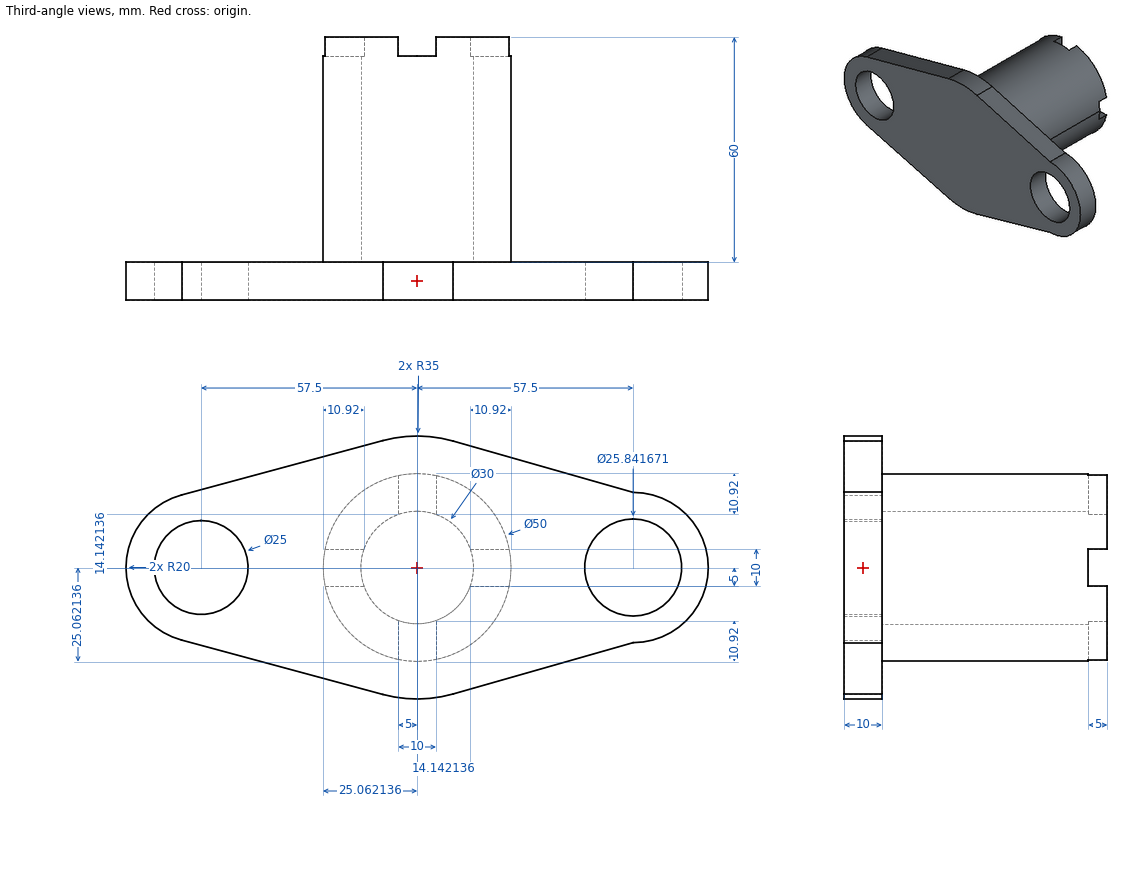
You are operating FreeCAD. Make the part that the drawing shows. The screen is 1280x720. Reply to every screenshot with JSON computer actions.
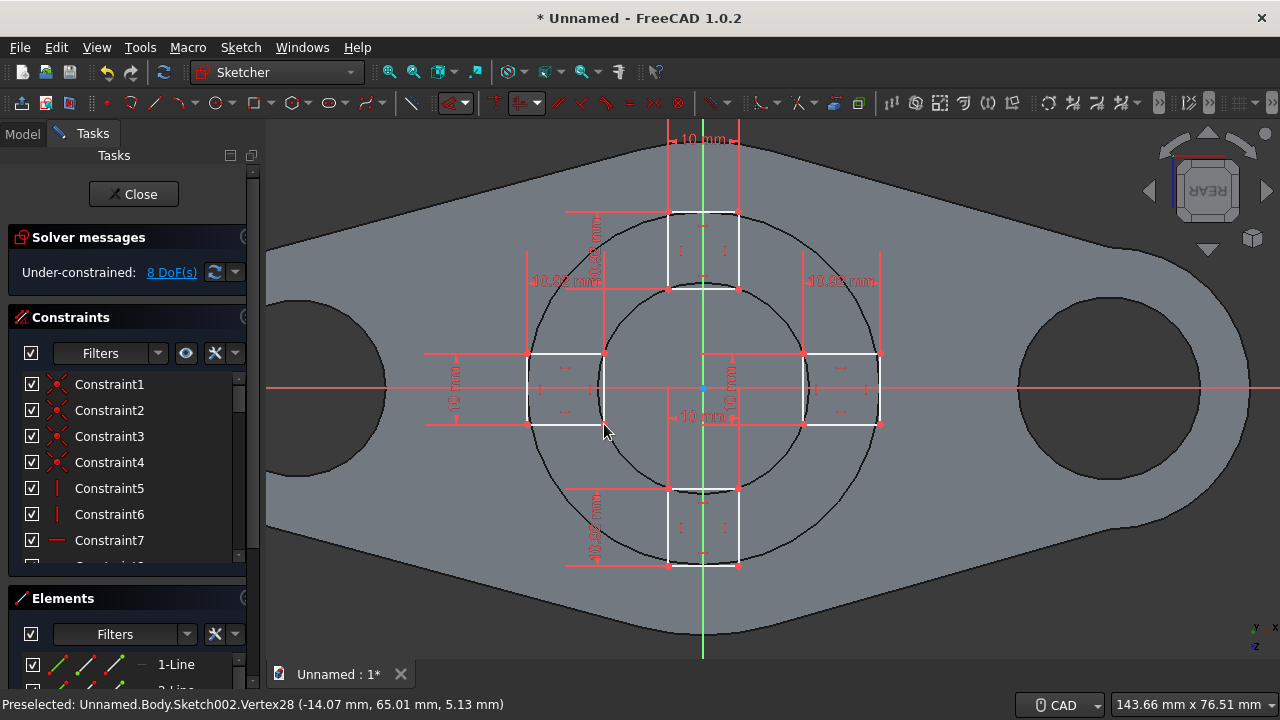
{"action": "left_click", "coordinate": [668, 212]}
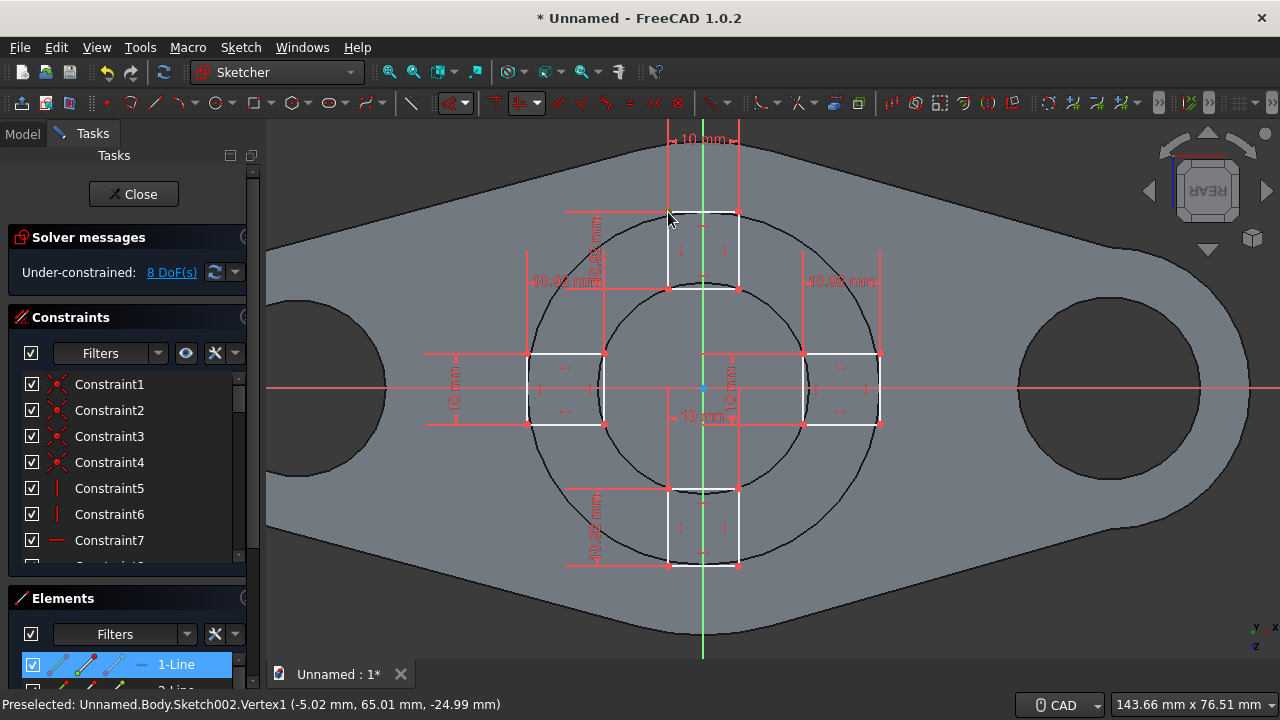
{"action": "left_click", "coordinate": [468, 104]}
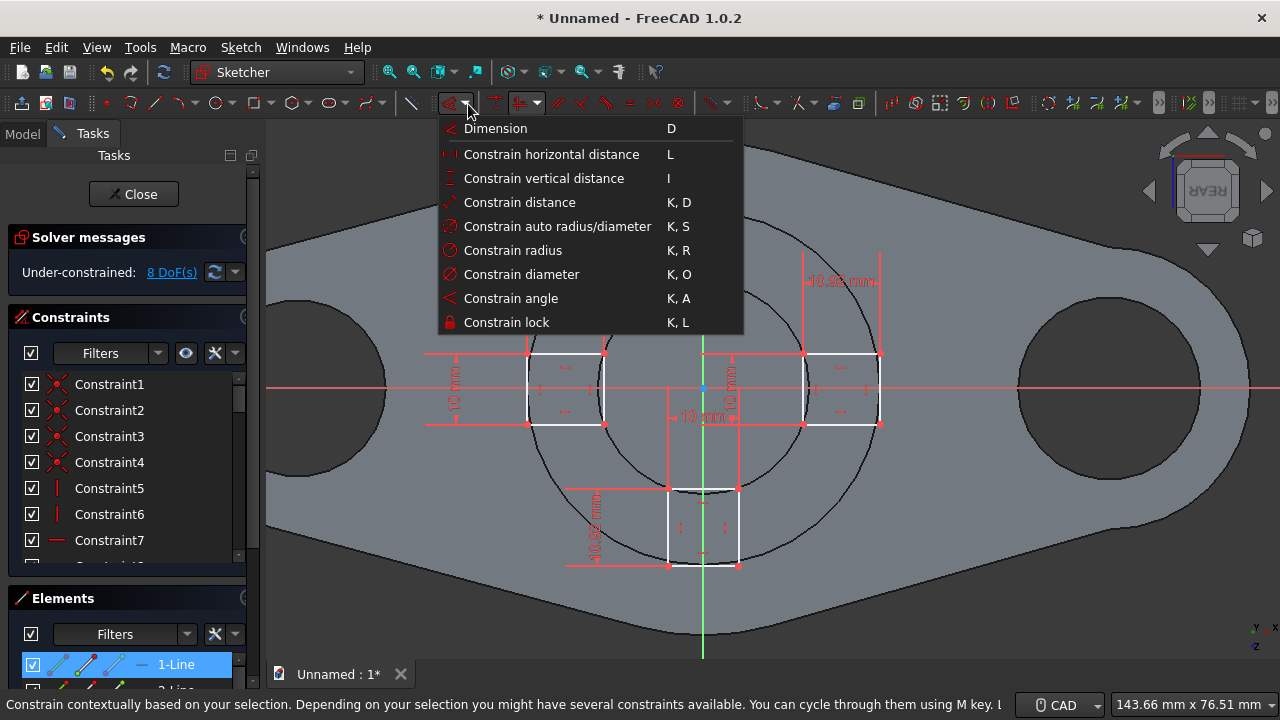
{"action": "left_click", "coordinate": [591, 154]}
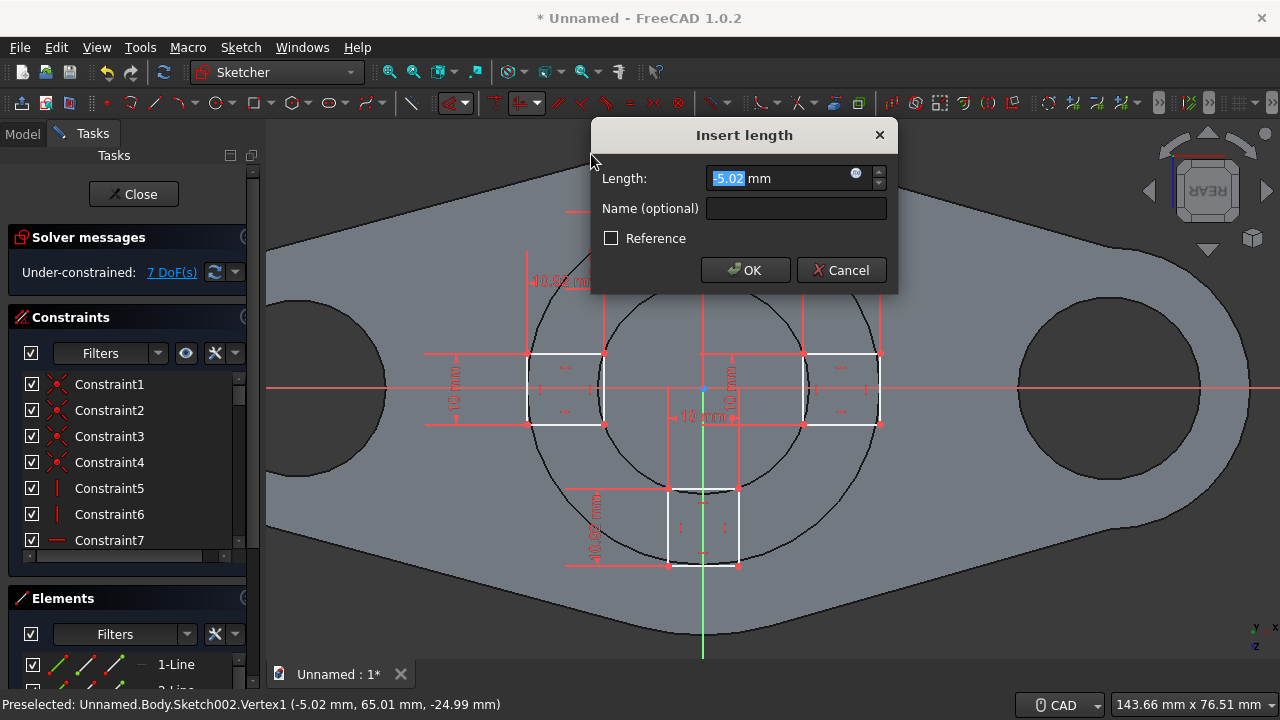
{"action": "type", "text": "-5"}
{"action": "key", "text": "Return"}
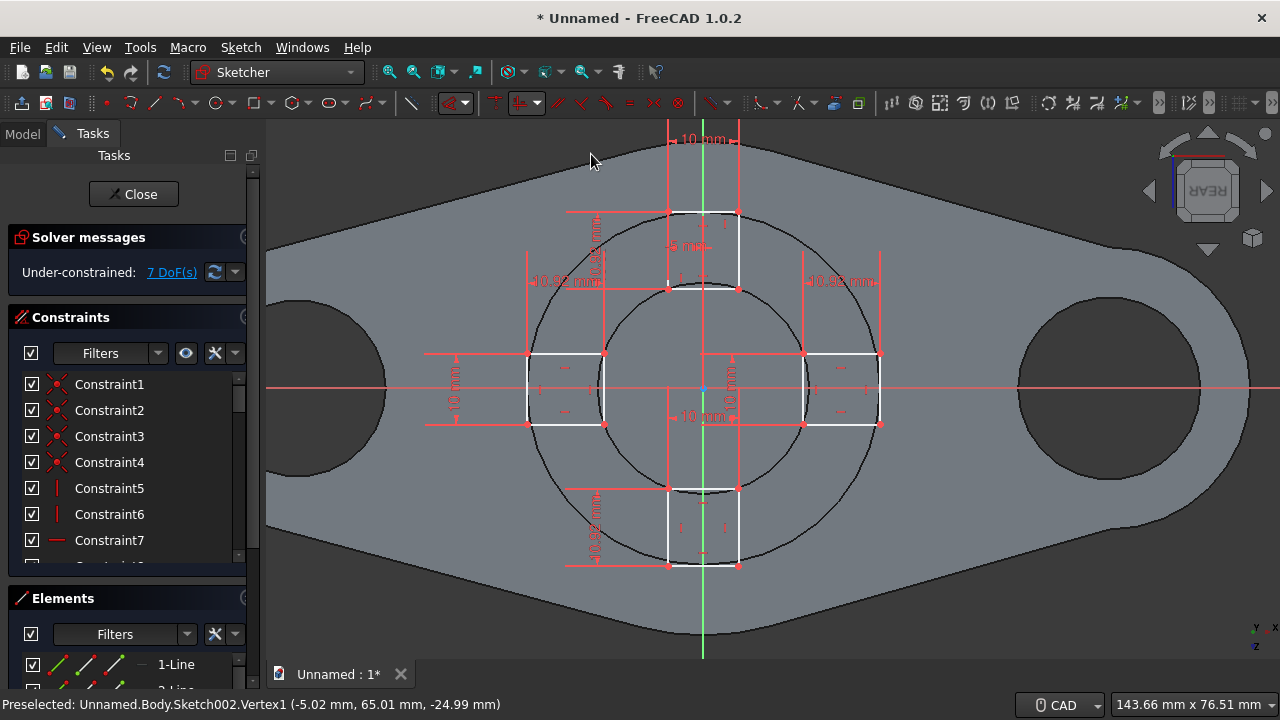
{"action": "left_click", "coordinate": [803, 354]}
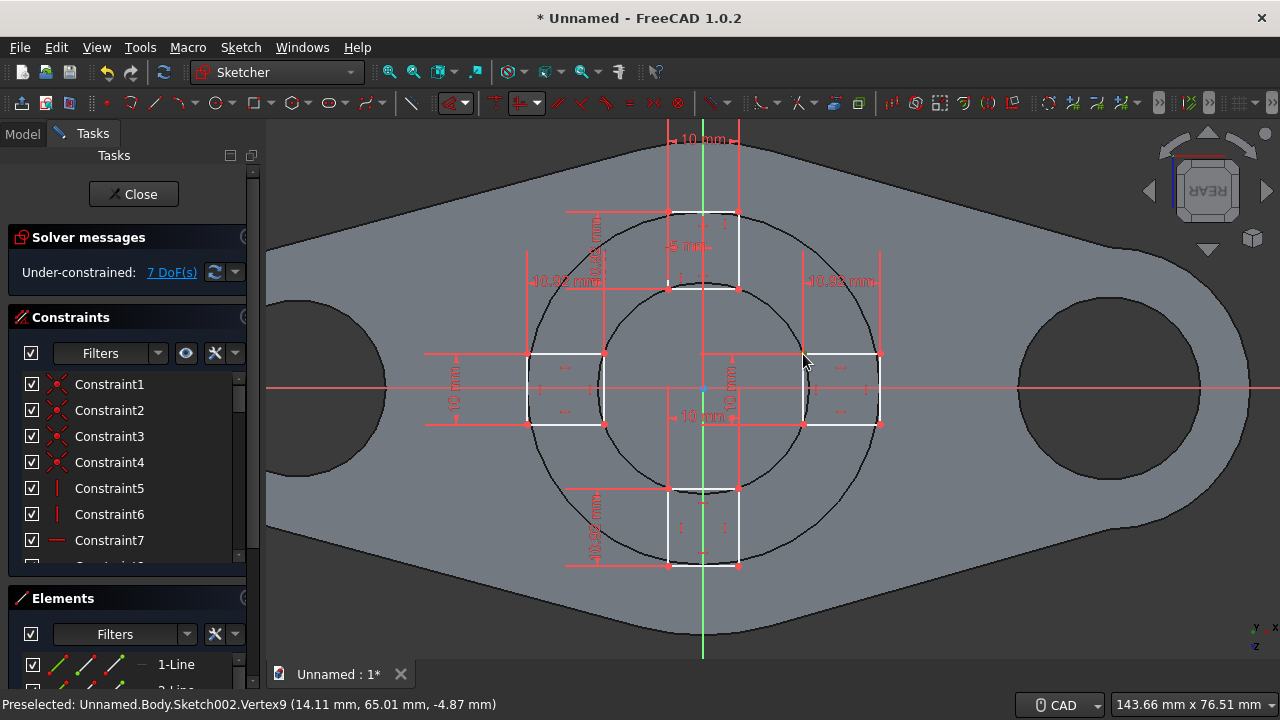
{"action": "key", "text": "i"}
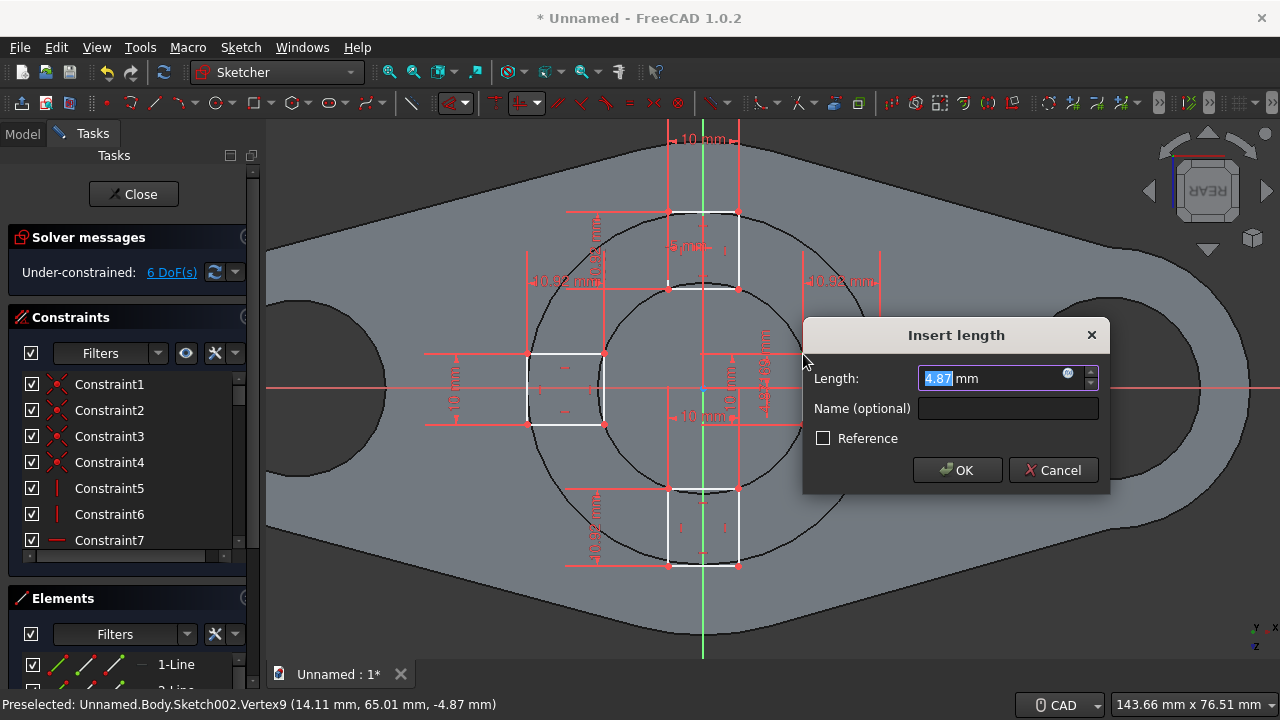
{"action": "type", "text": "5"}
{"action": "key", "text": "Return"}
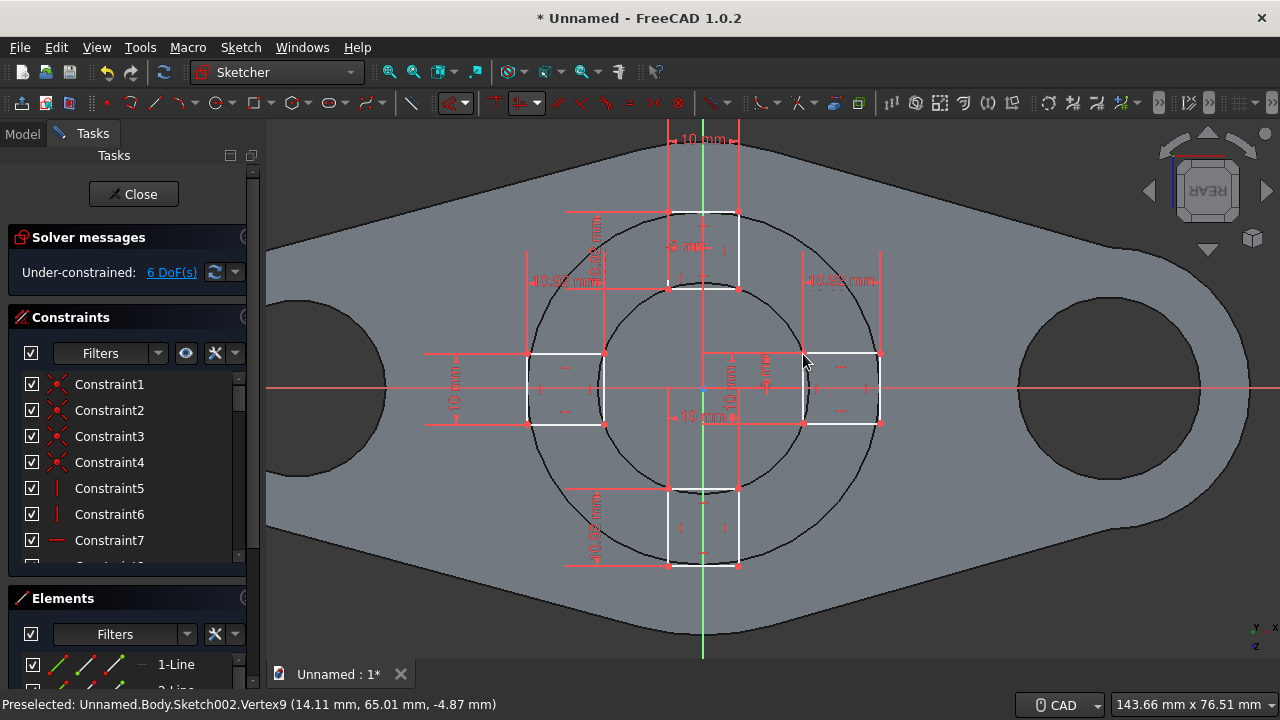
{"action": "left_click", "coordinate": [668, 489]}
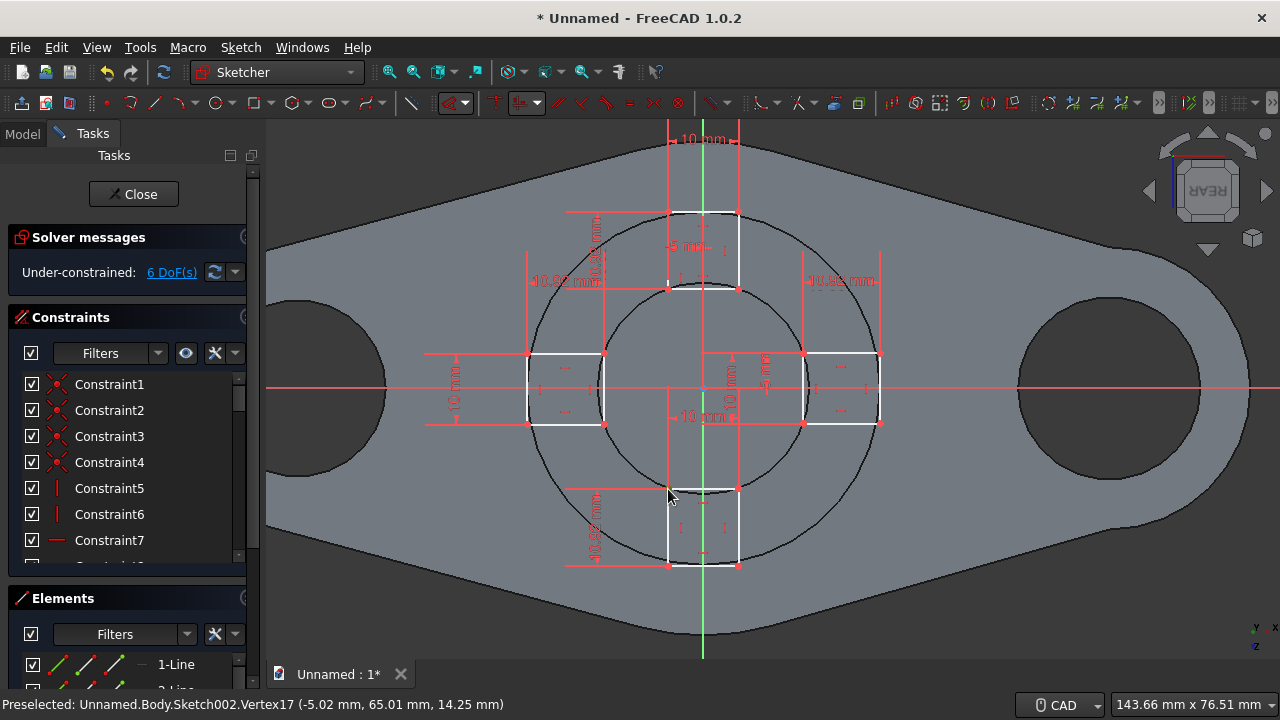
{"action": "key", "text": "l"}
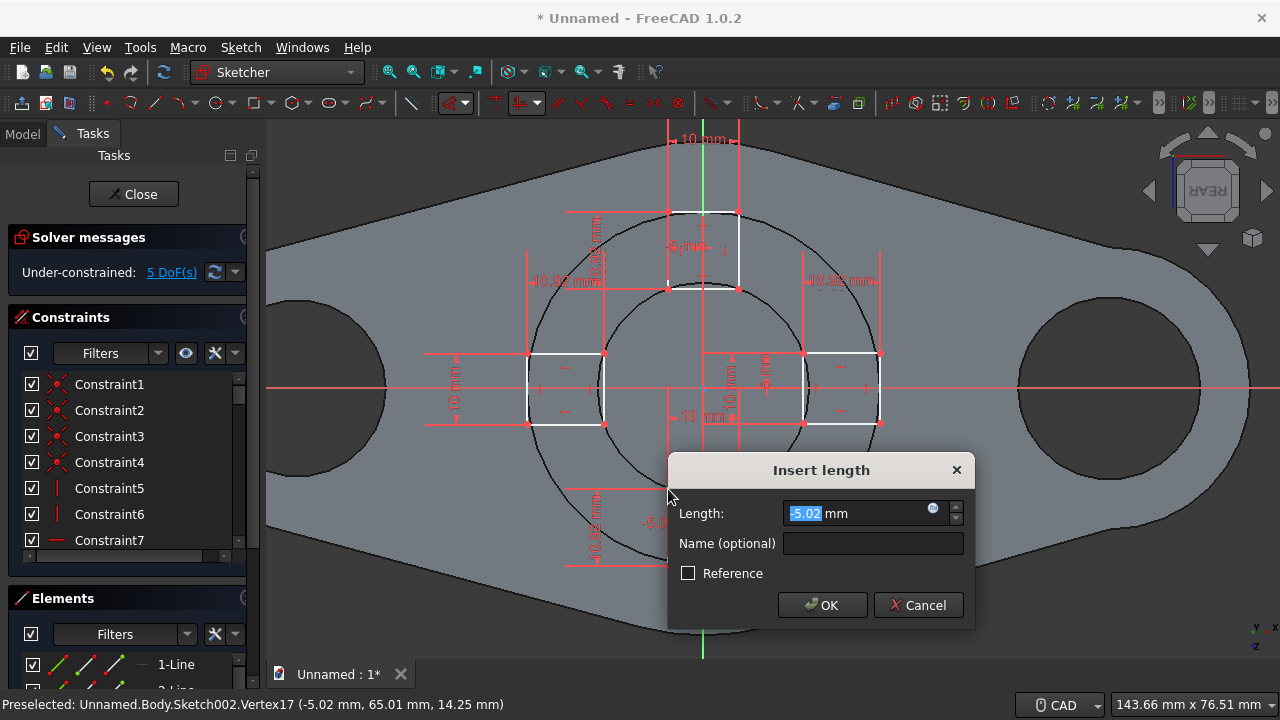
{"action": "type", "text": "-5"}
{"action": "key", "text": "Return"}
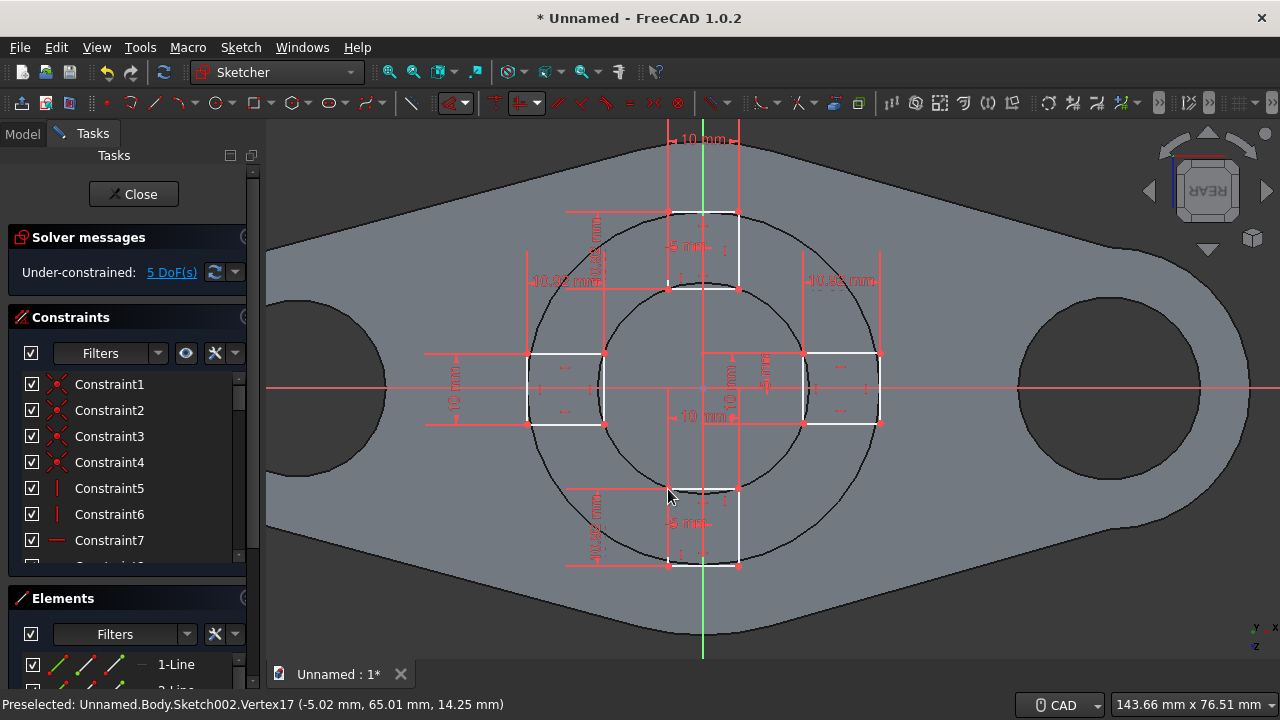
{"action": "left_click", "coordinate": [527, 354]}